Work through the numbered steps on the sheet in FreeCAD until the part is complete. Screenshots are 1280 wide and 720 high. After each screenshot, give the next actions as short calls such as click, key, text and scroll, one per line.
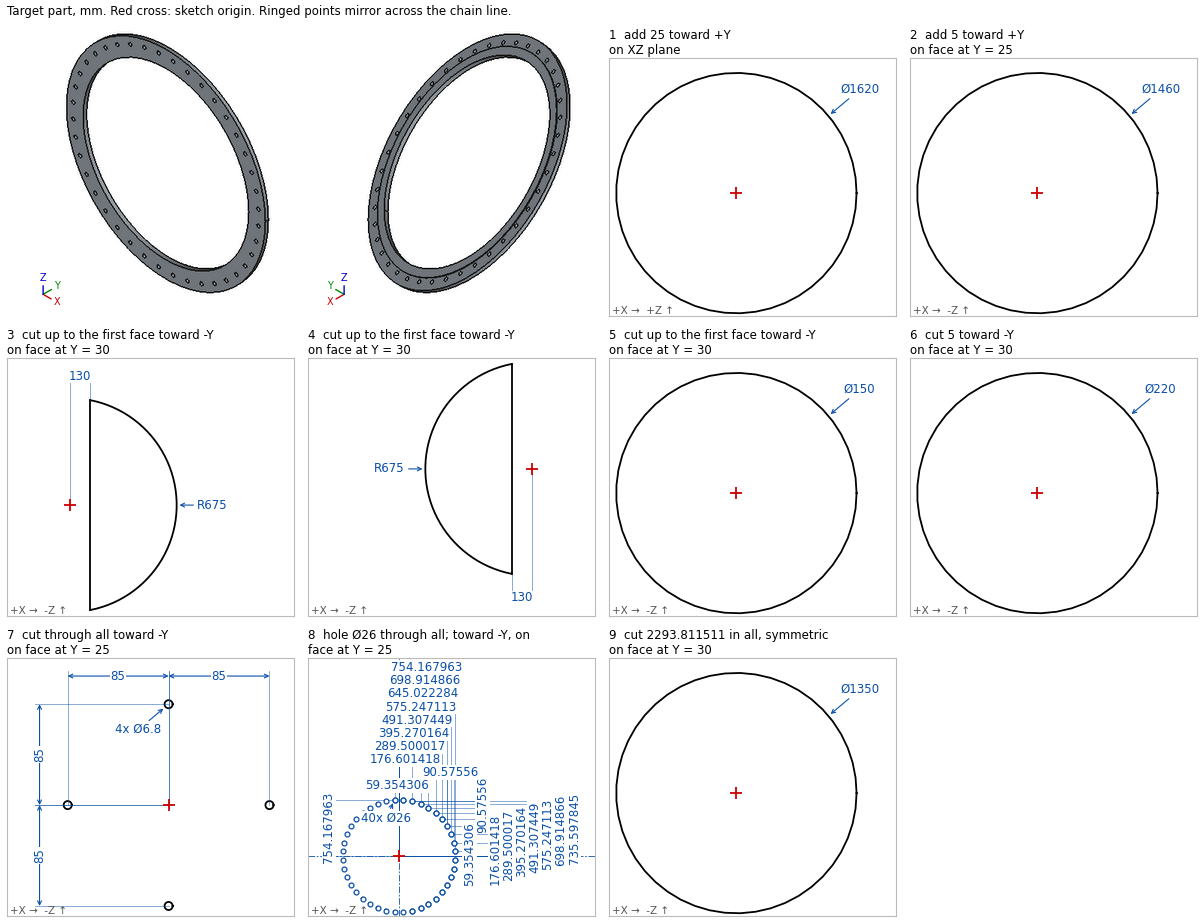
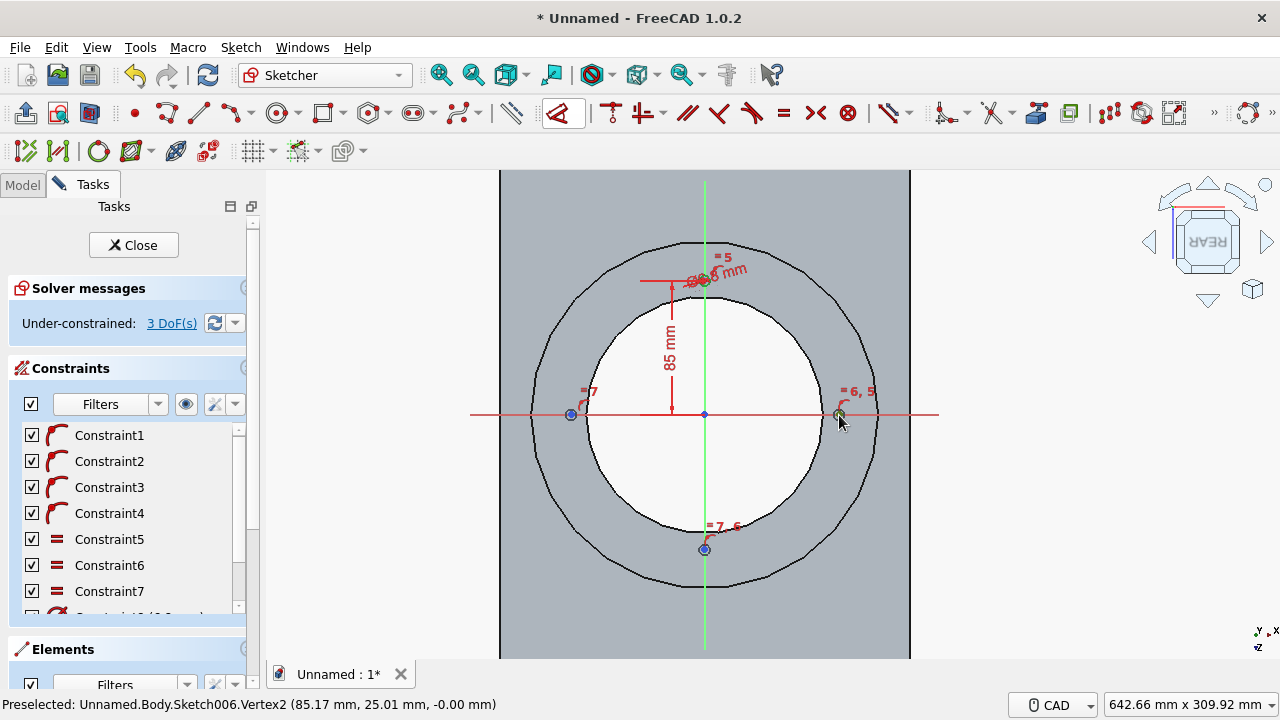
click(580, 114)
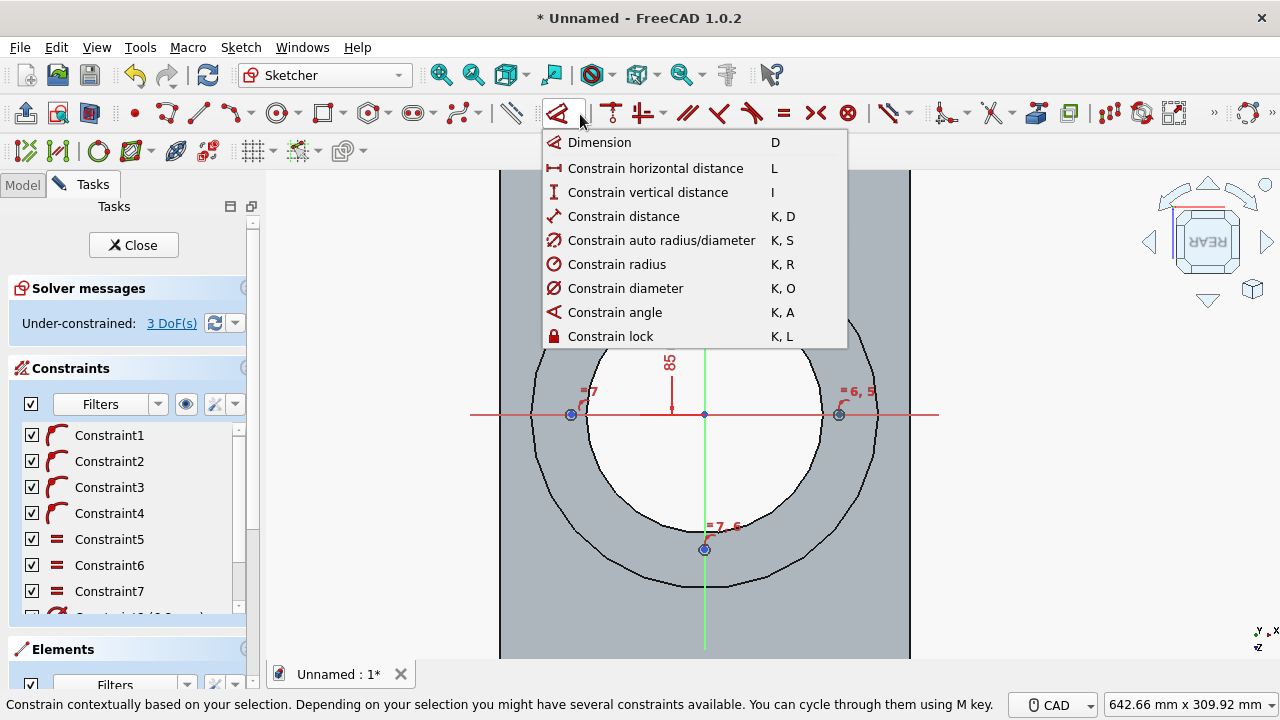
click(695, 168)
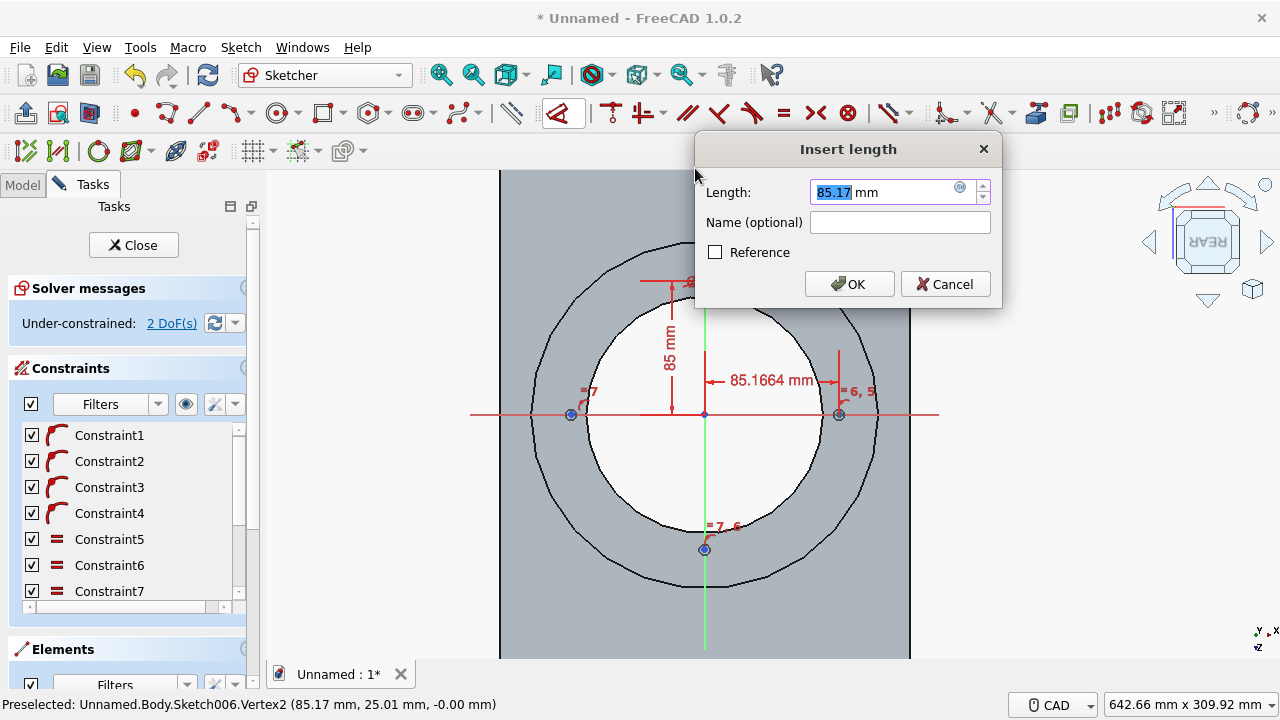
text(85)
key(Return)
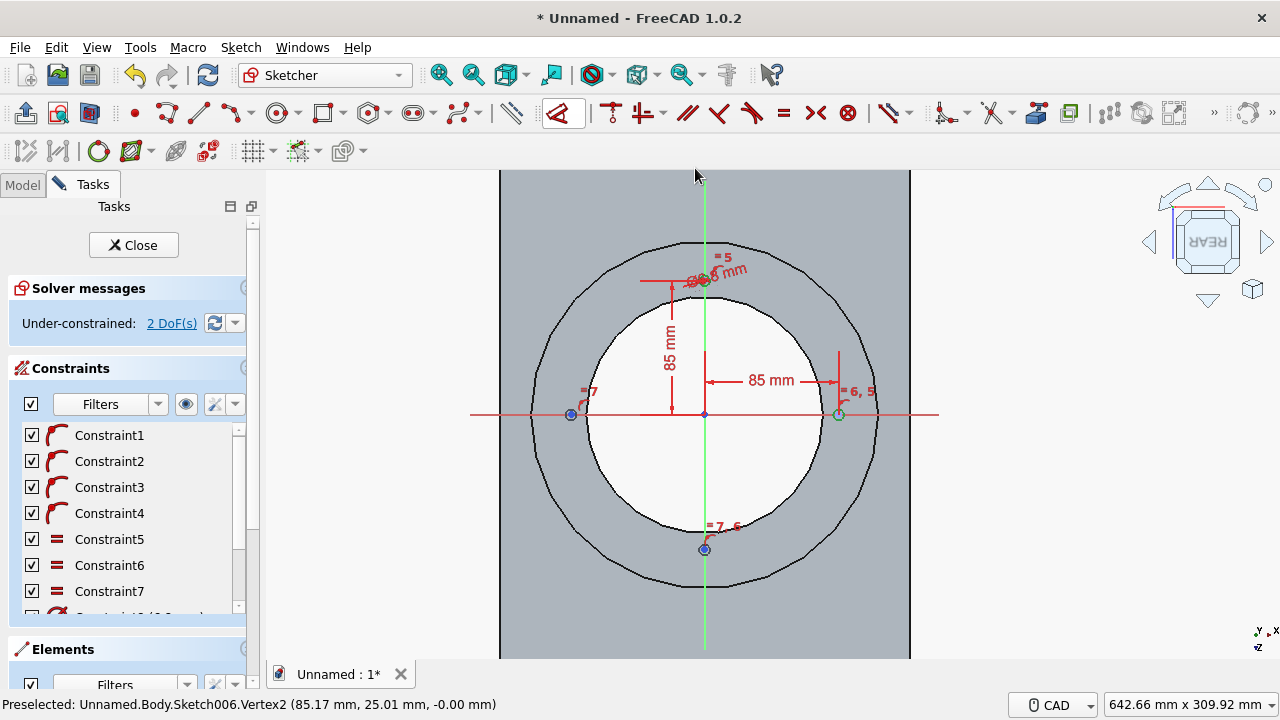
click(705, 550)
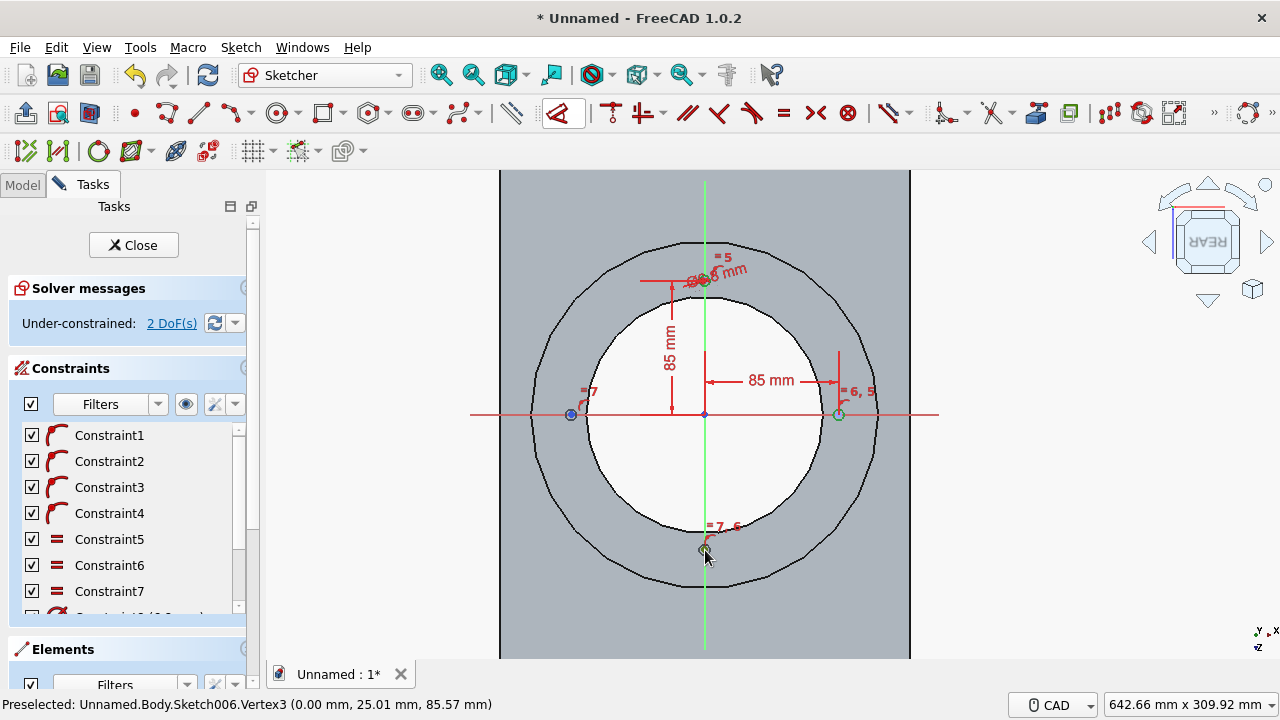
click(580, 114)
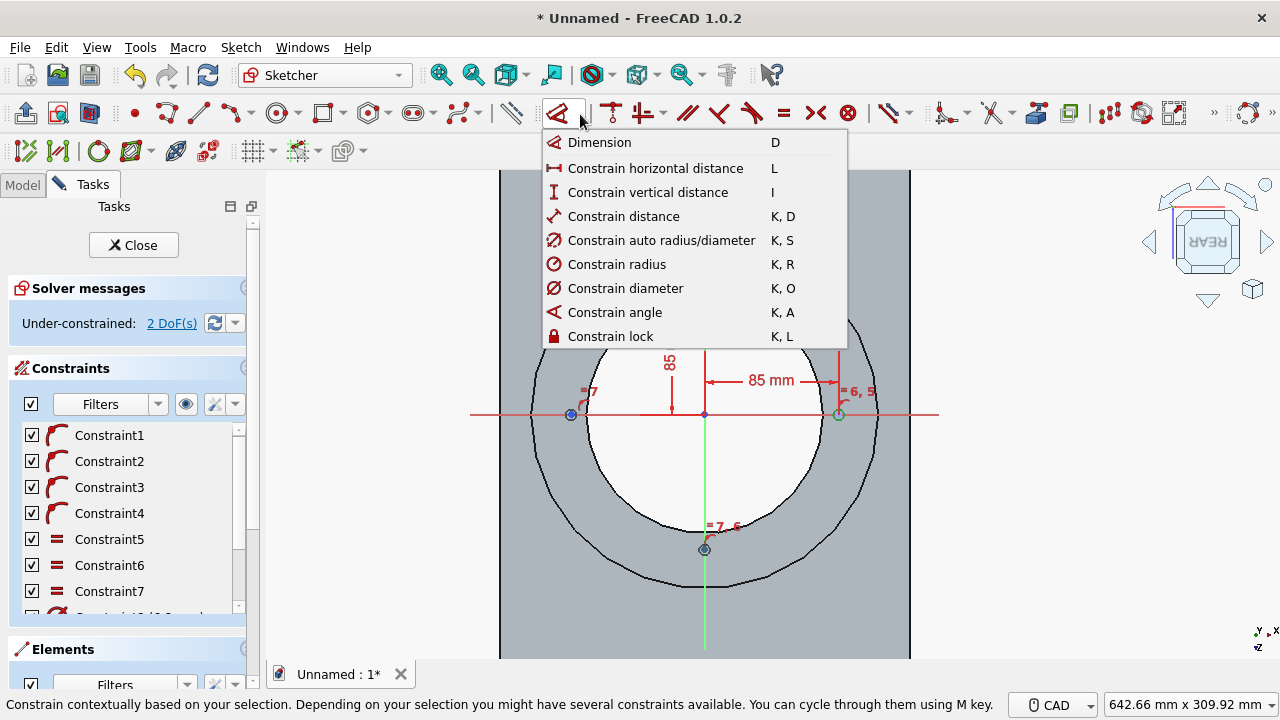
click(695, 192)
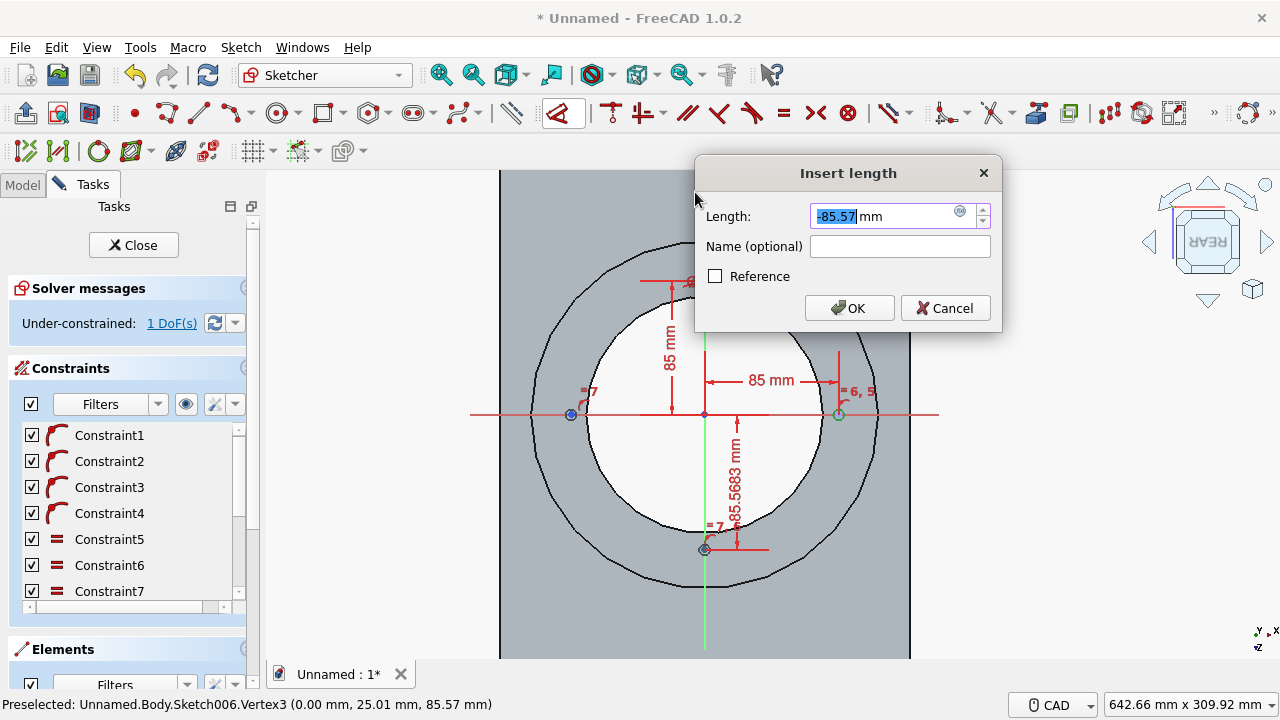
text(-85)
key(Return)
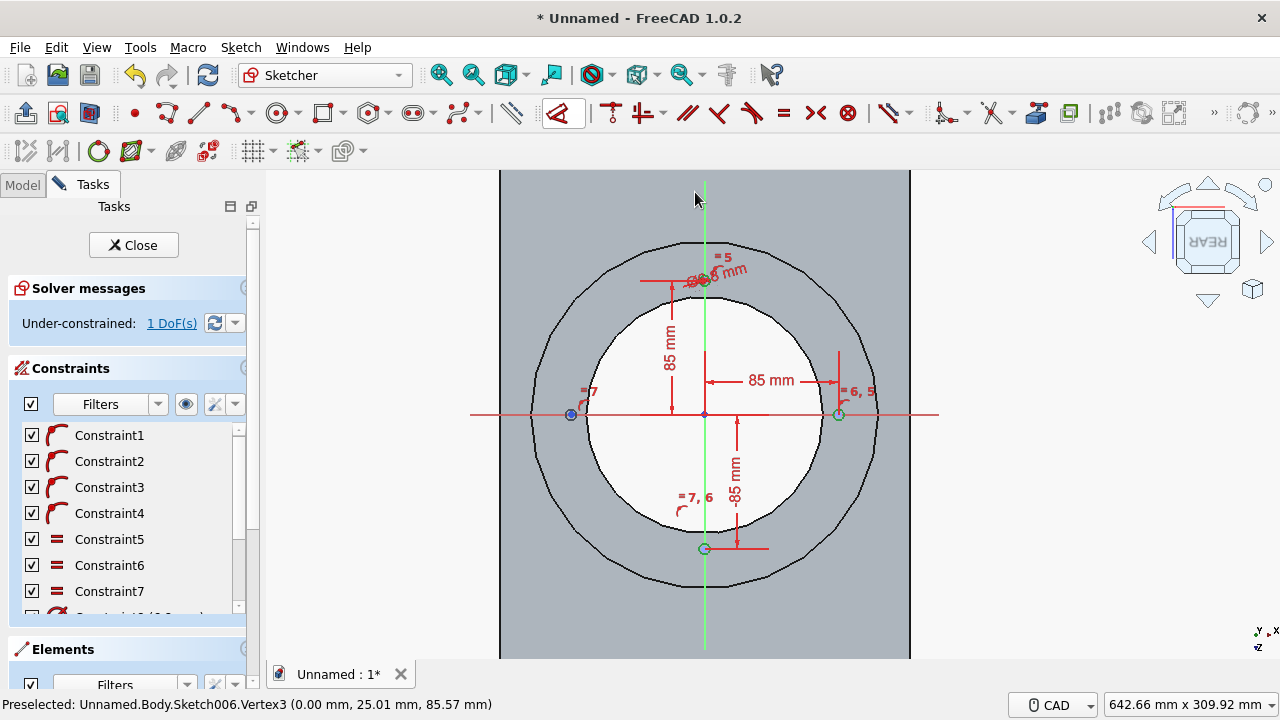
click(571, 415)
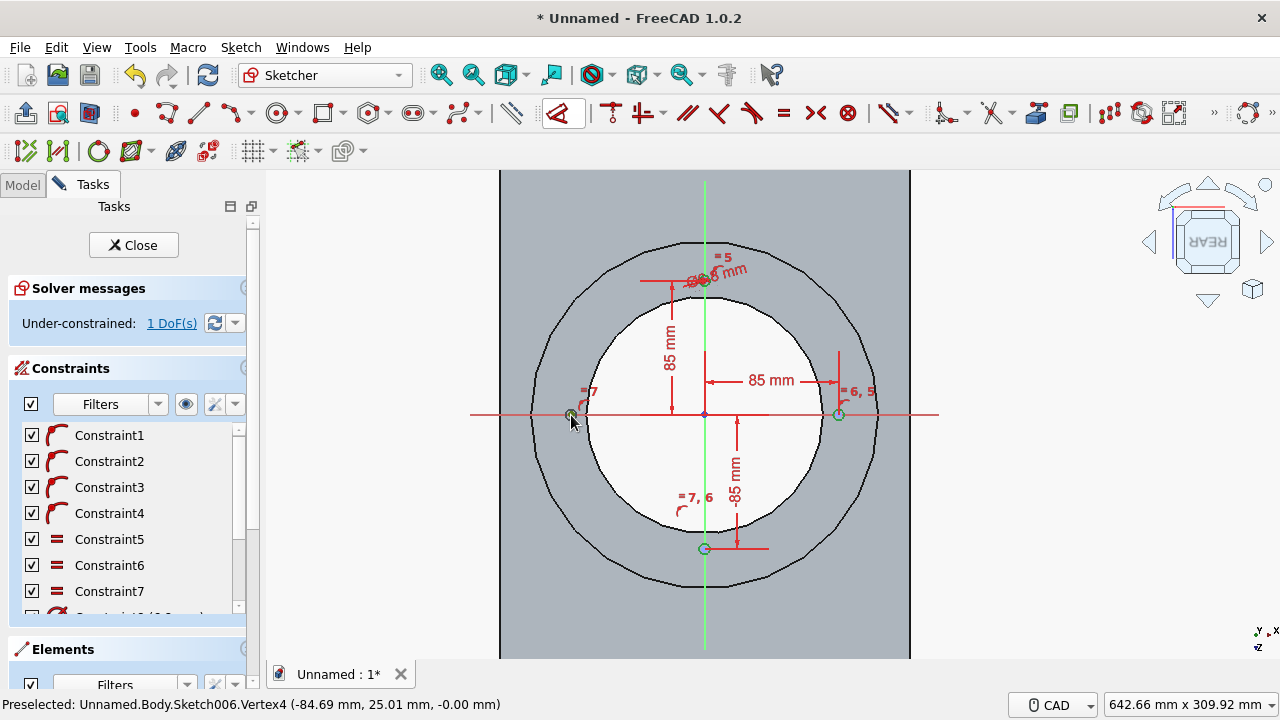
key(l)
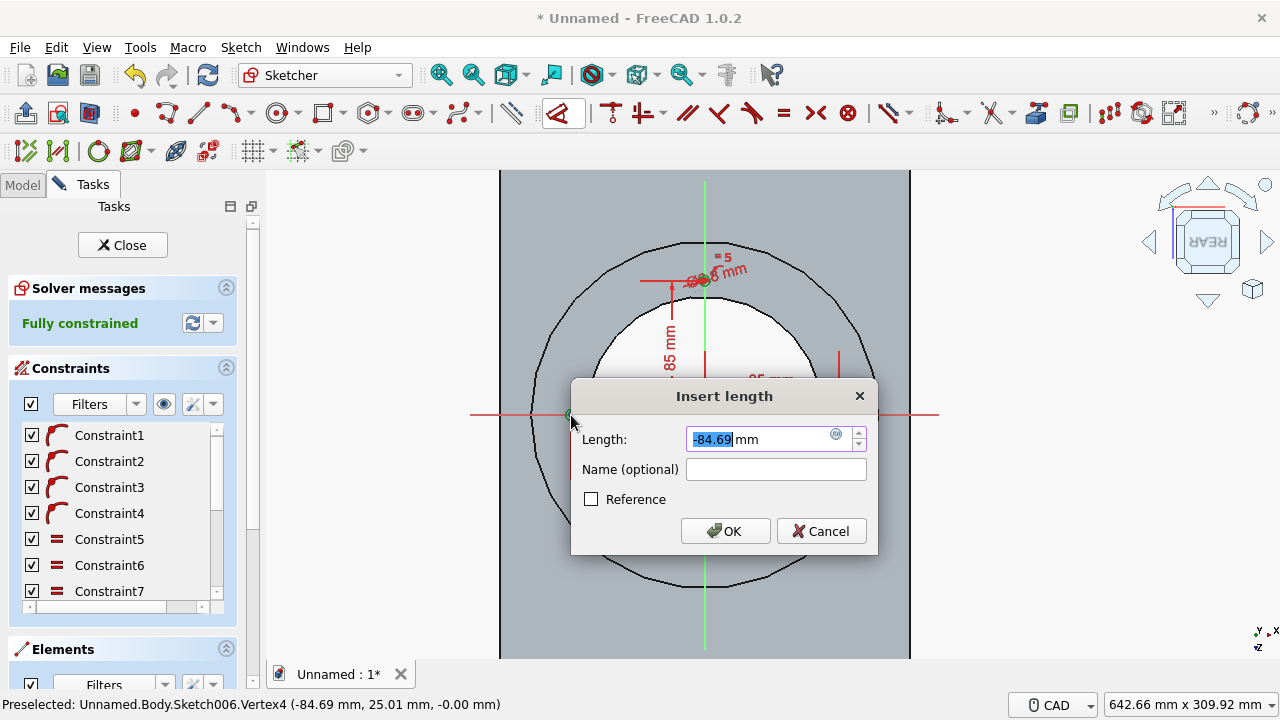
text(-85)
key(Return)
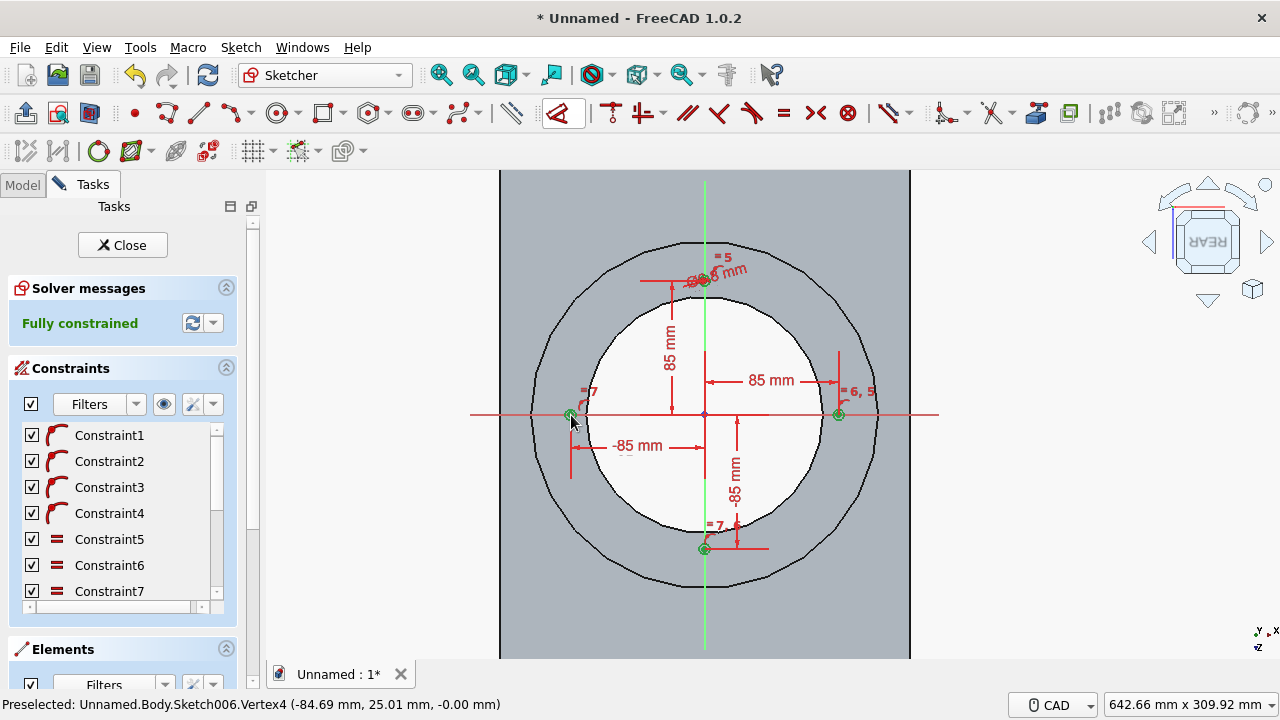
click(123, 245)